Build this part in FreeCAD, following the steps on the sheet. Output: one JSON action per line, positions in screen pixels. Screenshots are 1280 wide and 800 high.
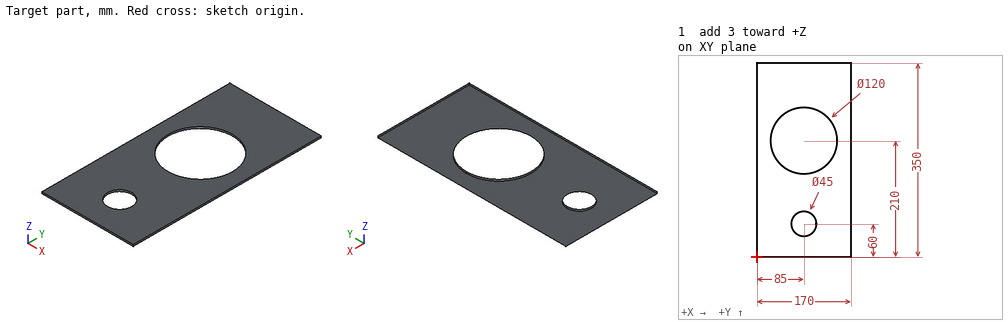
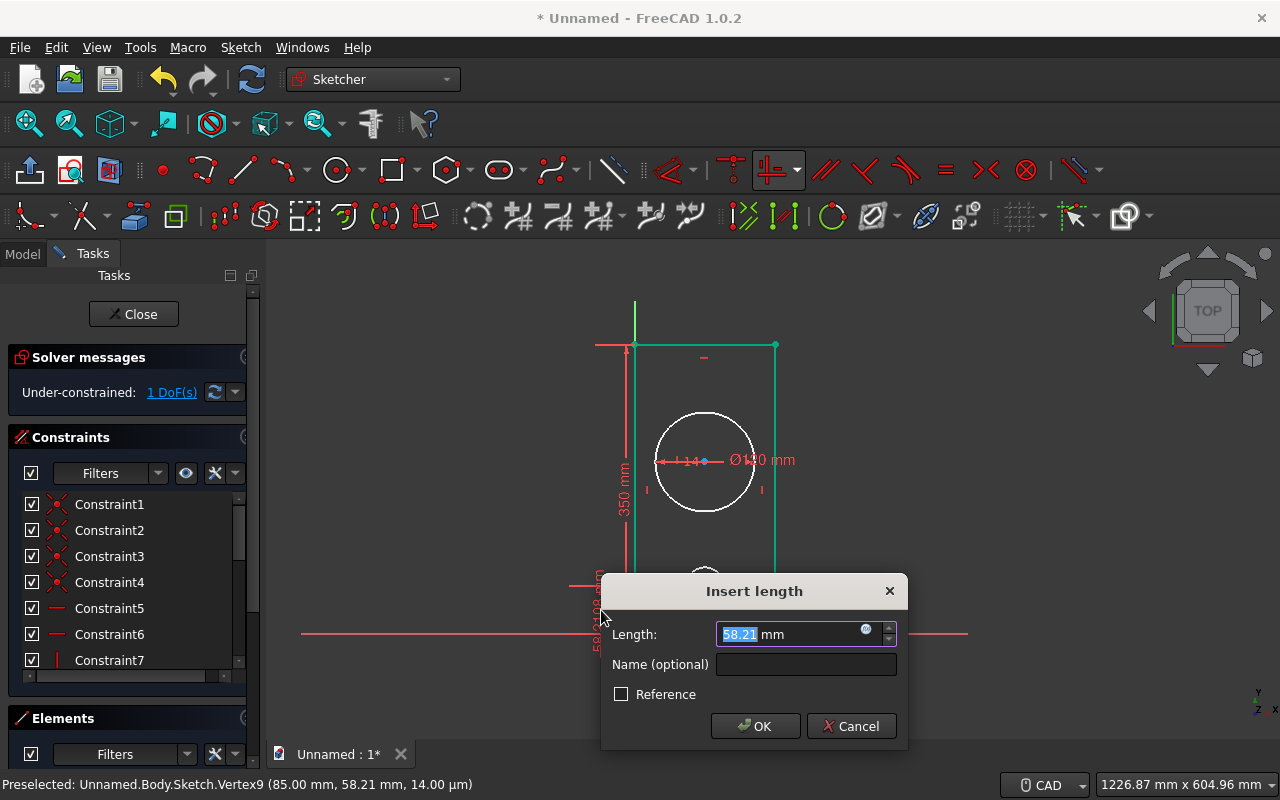
{"action": "type", "text": "60"}
{"action": "key", "text": "Return"}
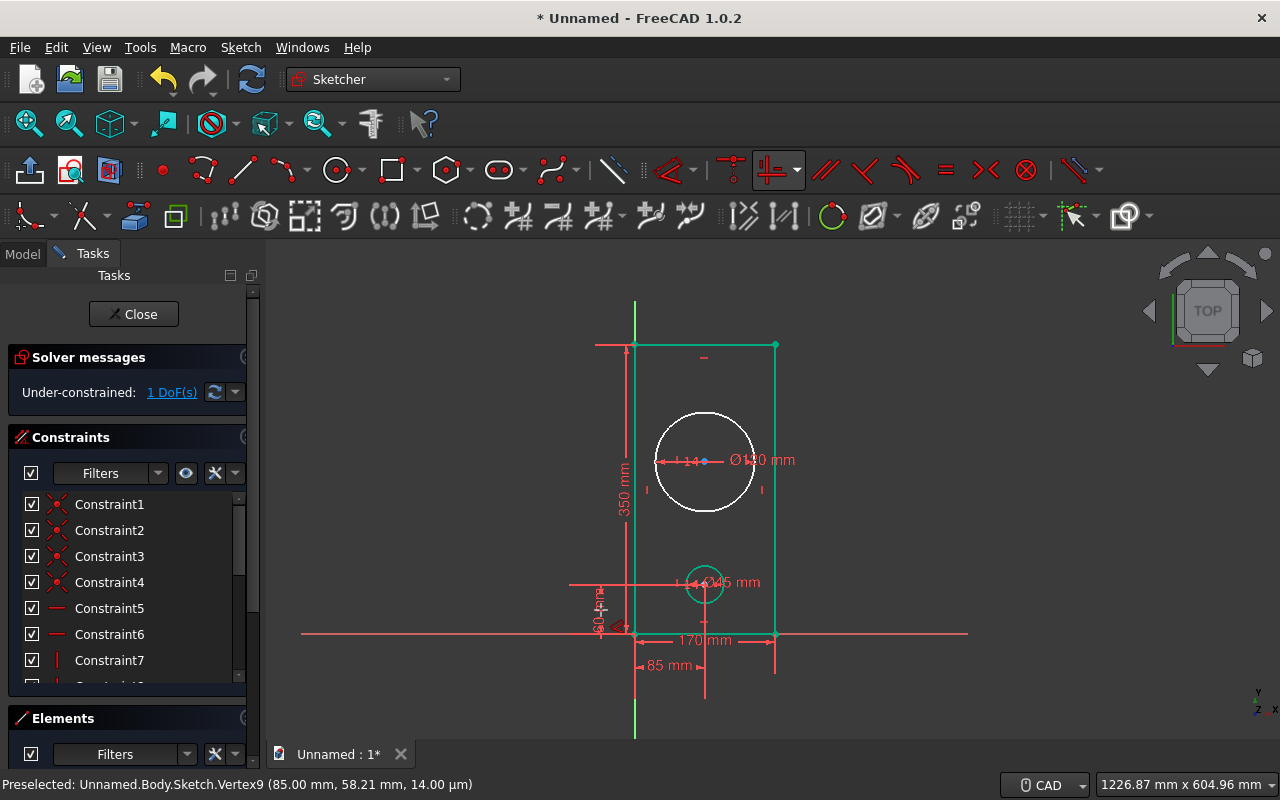
{"action": "left_click", "coordinate": [705, 462]}
{"action": "left_click", "coordinate": [601, 548]}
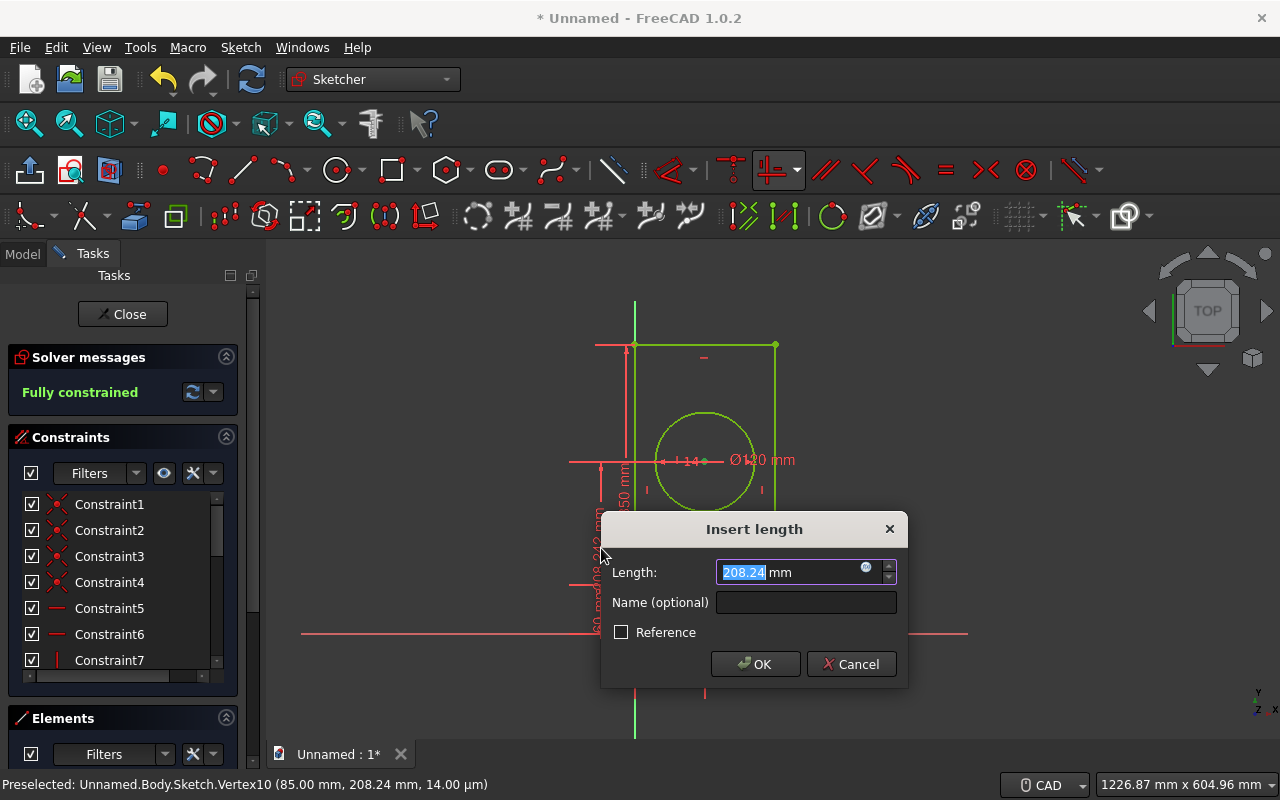
{"action": "type", "text": "210"}
{"action": "key", "text": "Return"}
{"action": "key", "text": "Escape"}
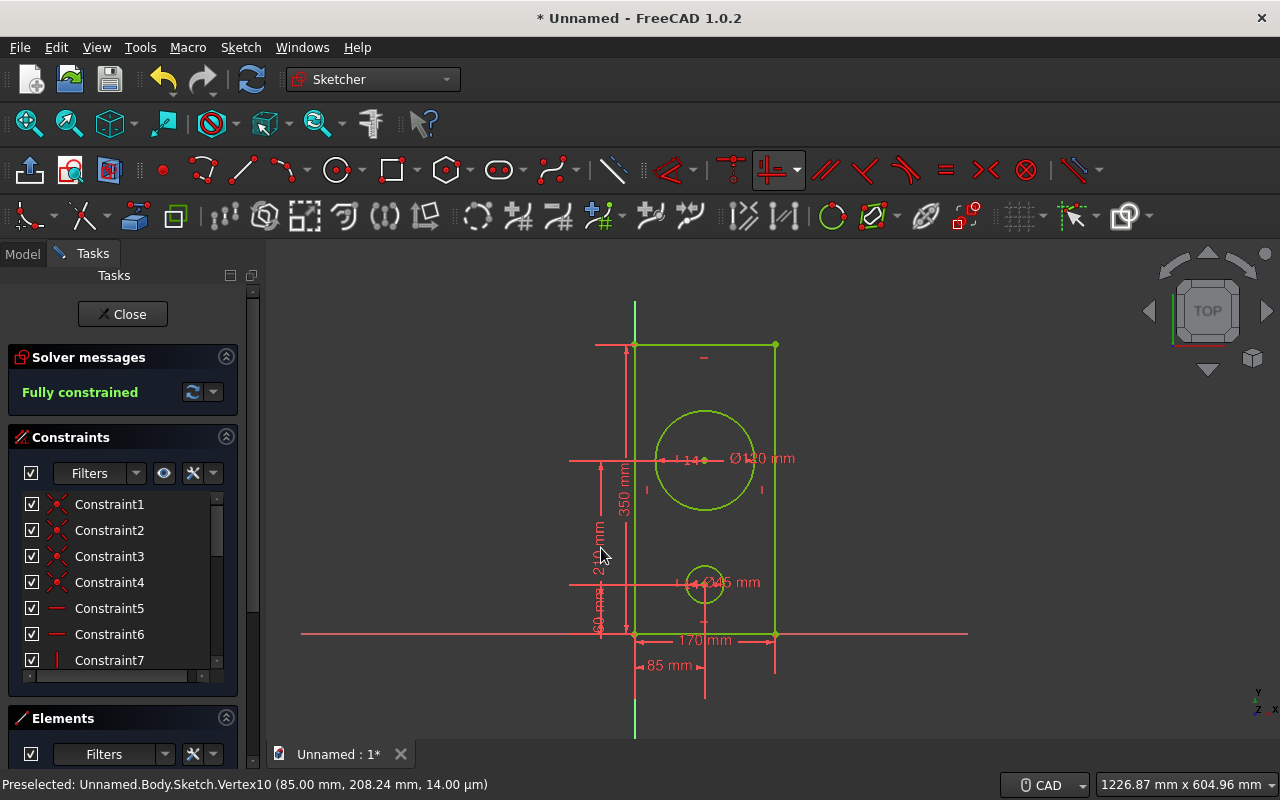
{"action": "left_click", "coordinate": [123, 314]}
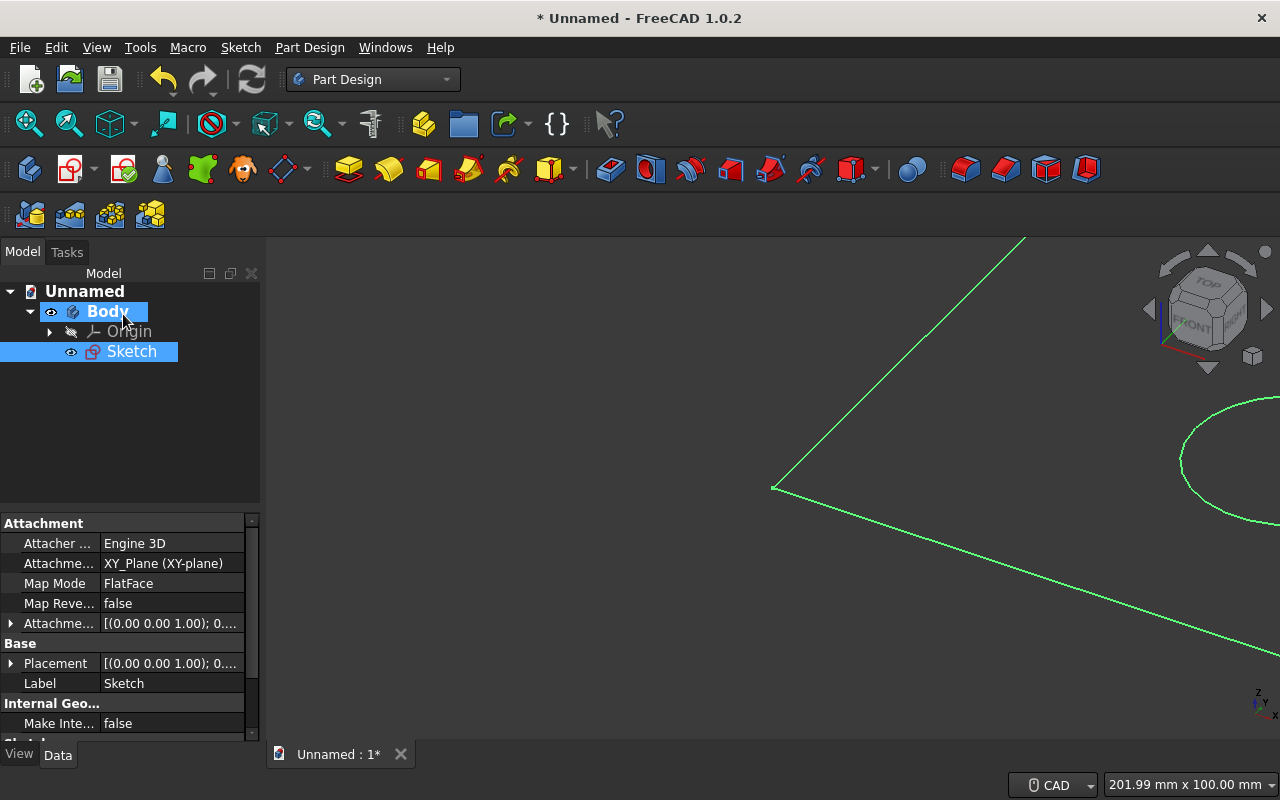
{"action": "left_click", "coordinate": [350, 170]}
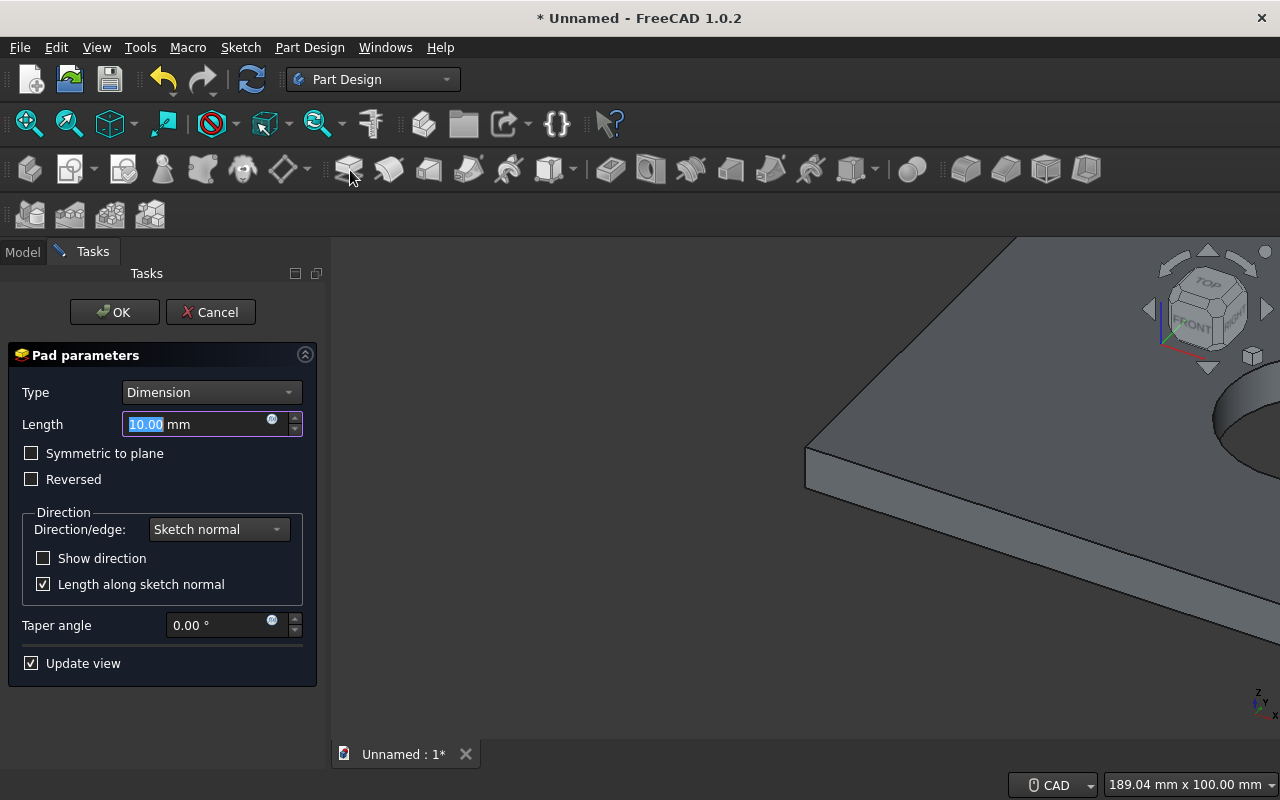
{"action": "type", "text": "3"}
{"action": "key", "text": "Tab"}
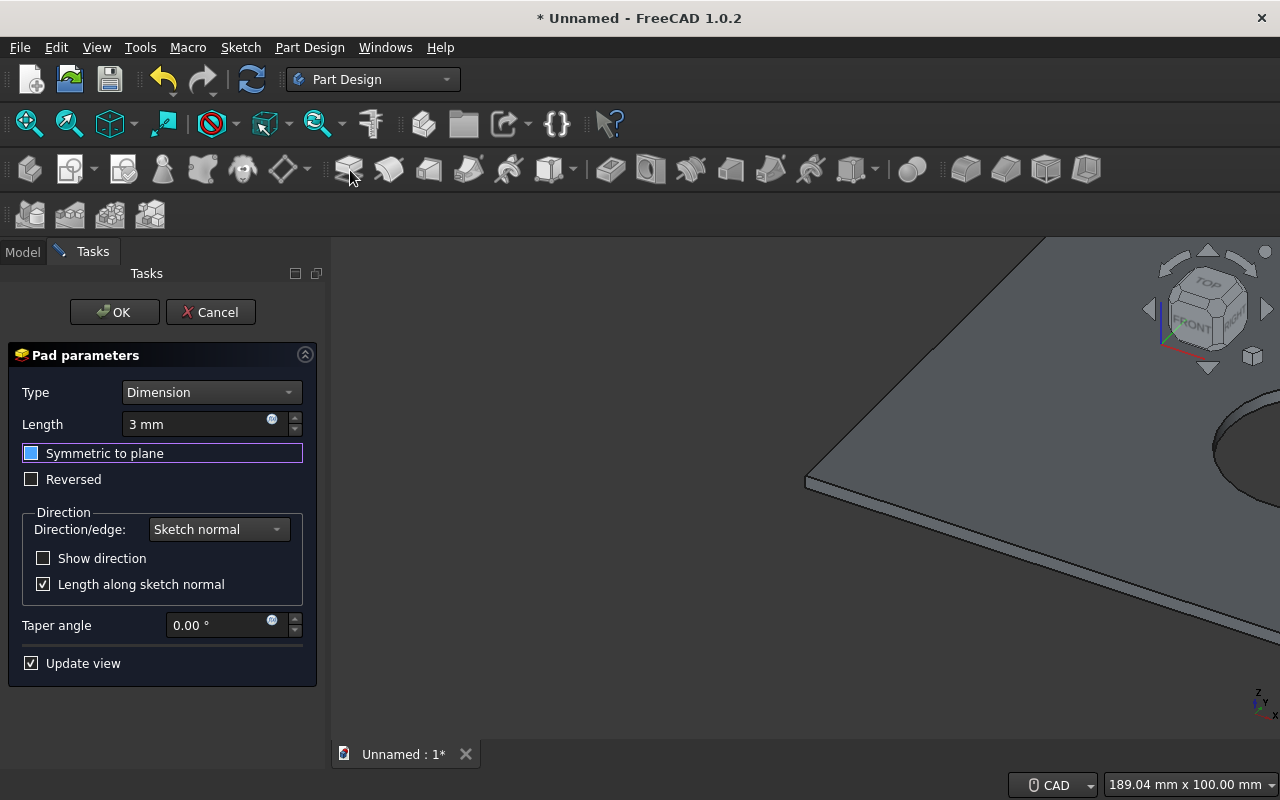
{"action": "left_click", "coordinate": [115, 312]}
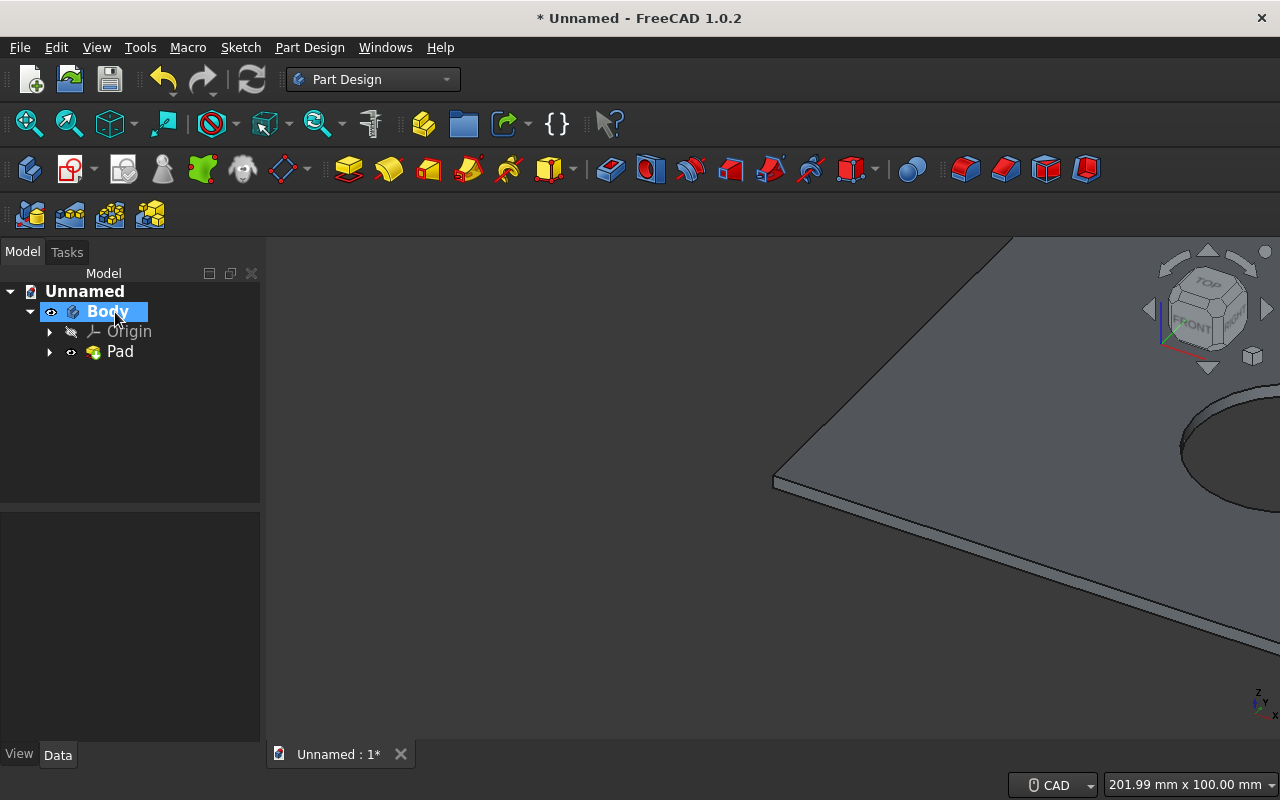
{"action": "key", "text": "0"}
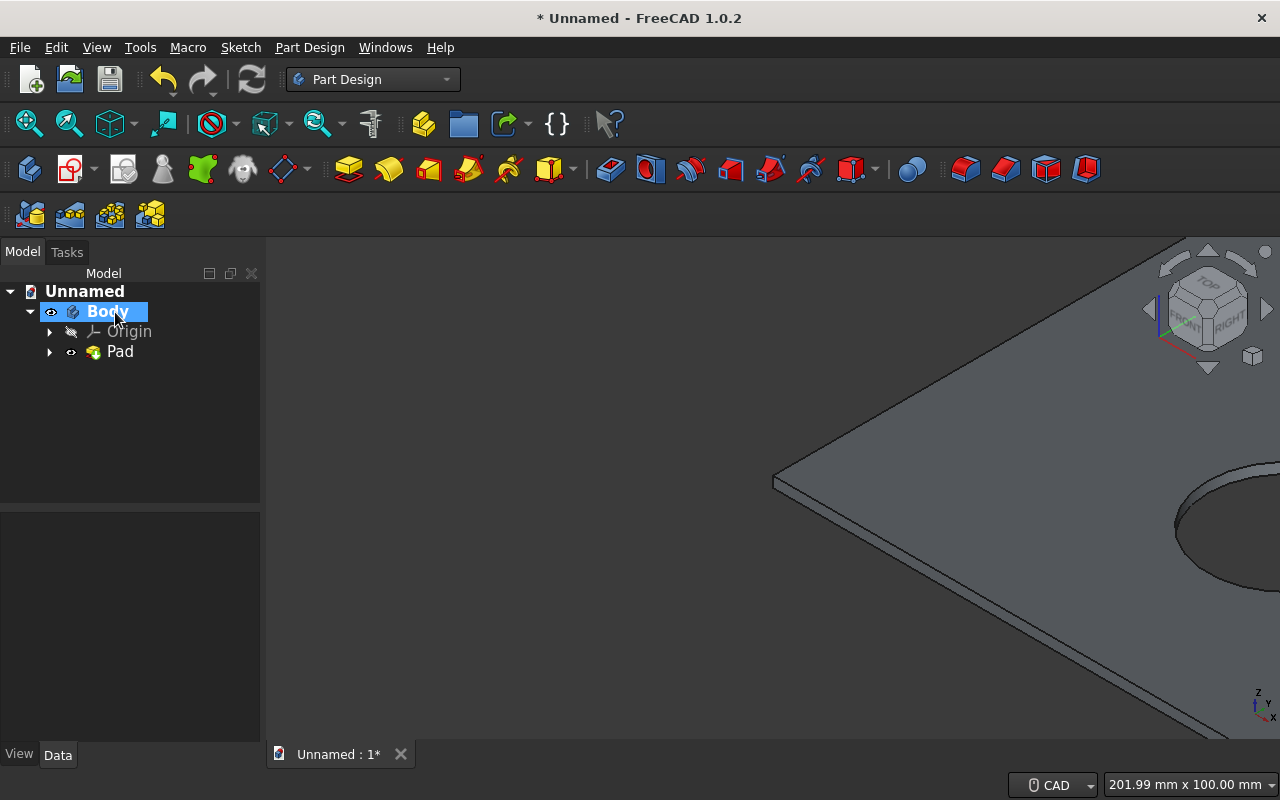
{"action": "left_click", "coordinate": [30, 124]}